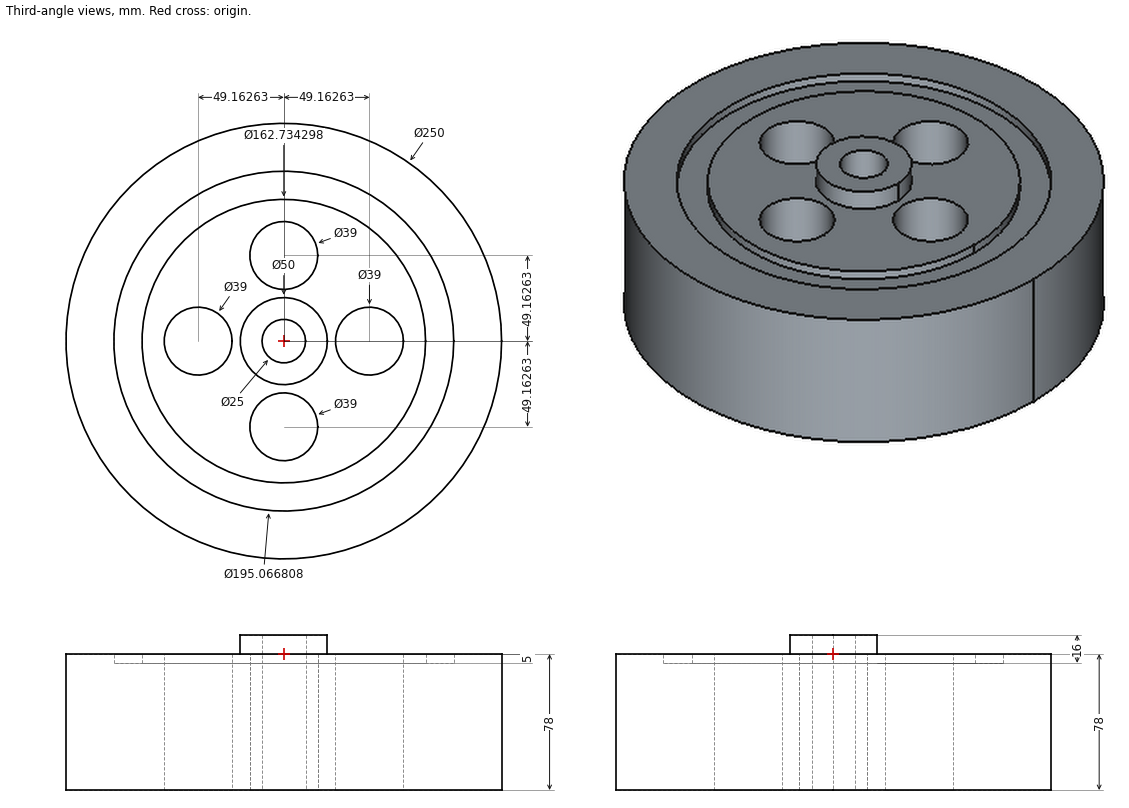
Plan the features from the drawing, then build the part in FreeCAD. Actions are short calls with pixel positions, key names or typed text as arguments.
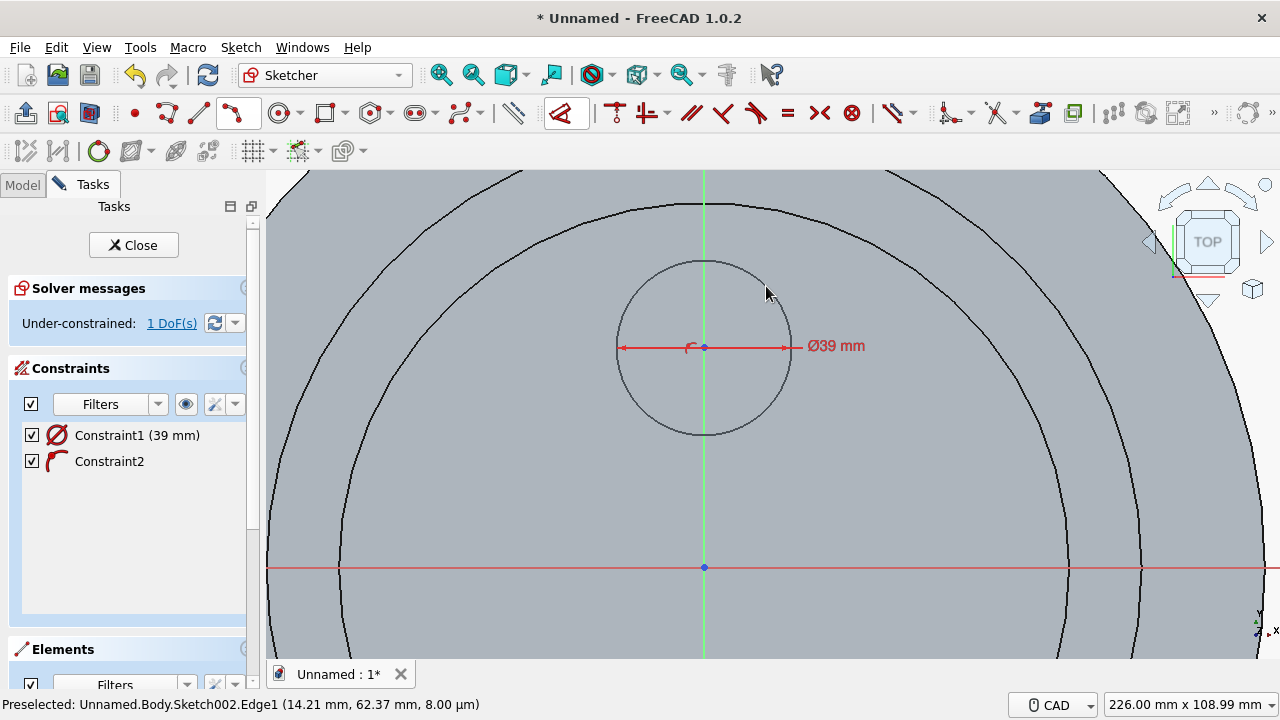
click(560, 114)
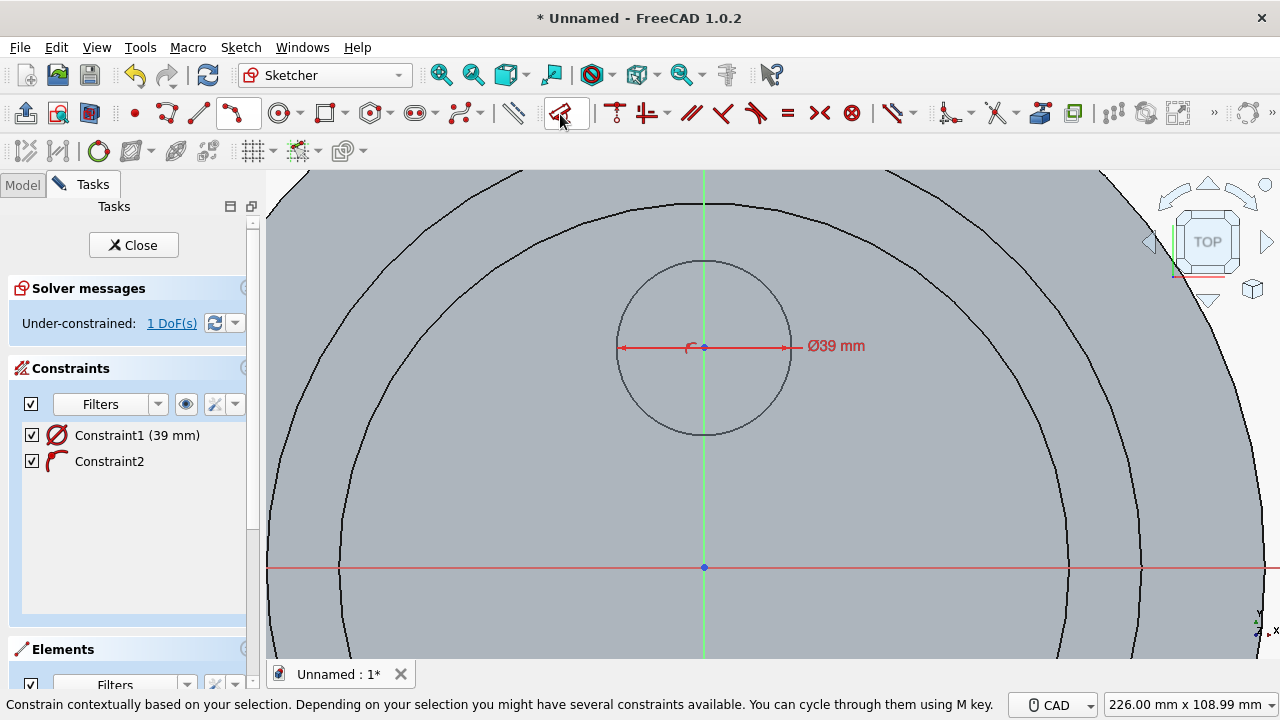
click(704, 348)
click(738, 458)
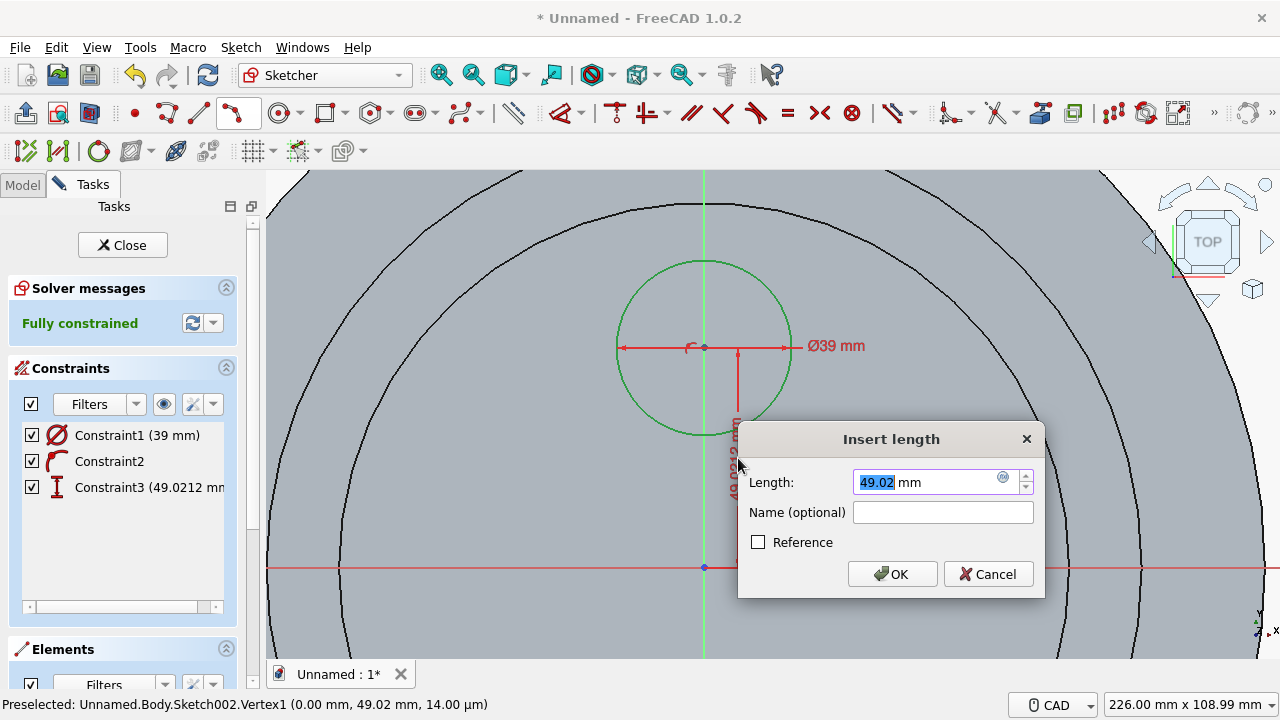
text(49.16263)
key(Return)
key(Escape)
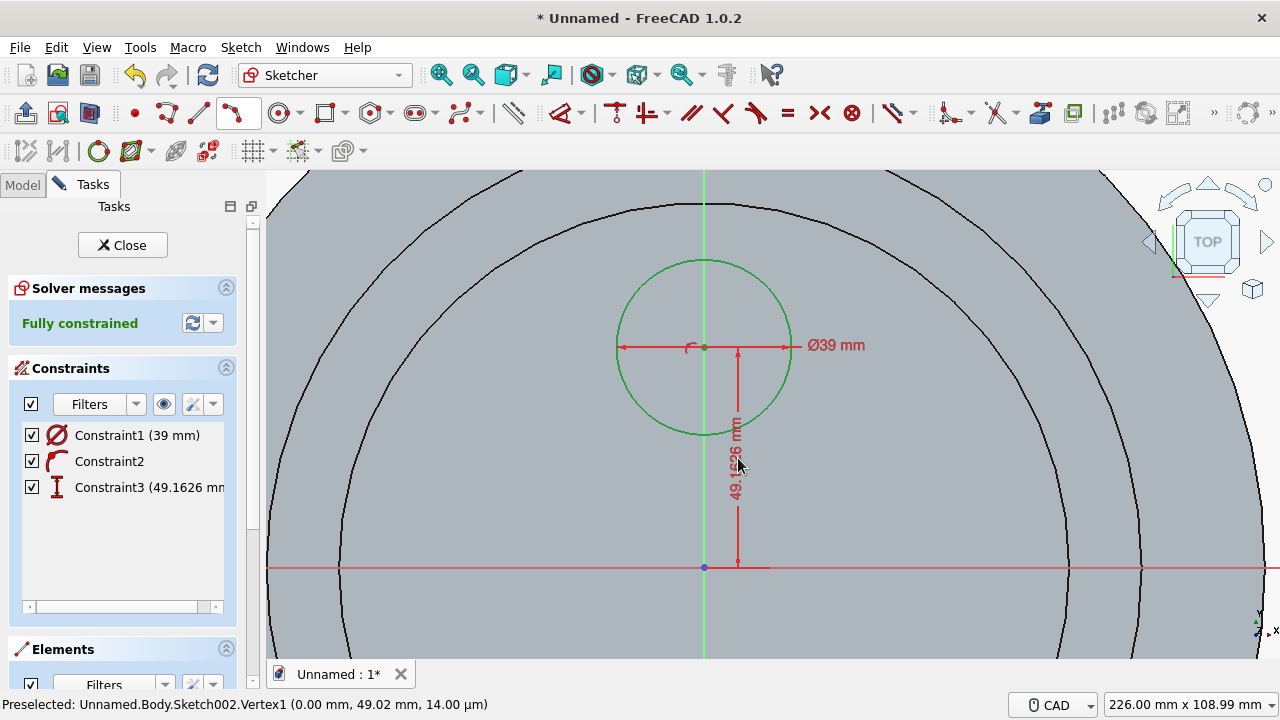
click(123, 245)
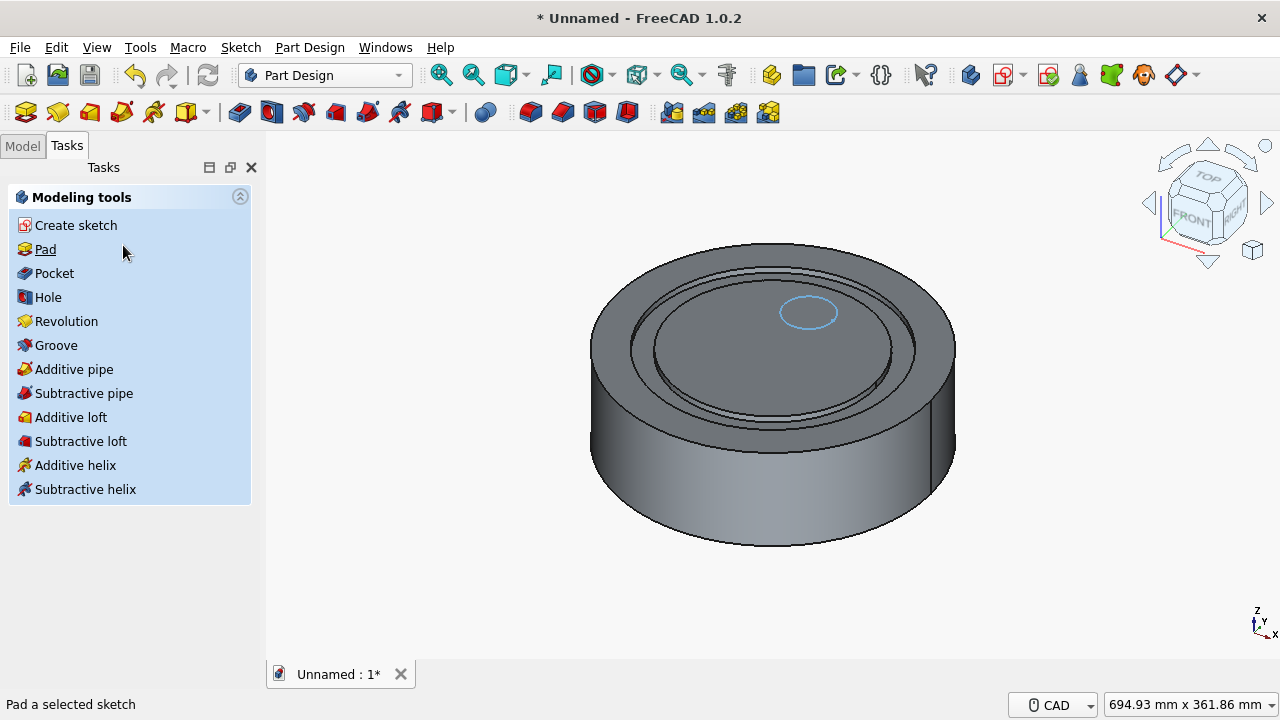
click(240, 112)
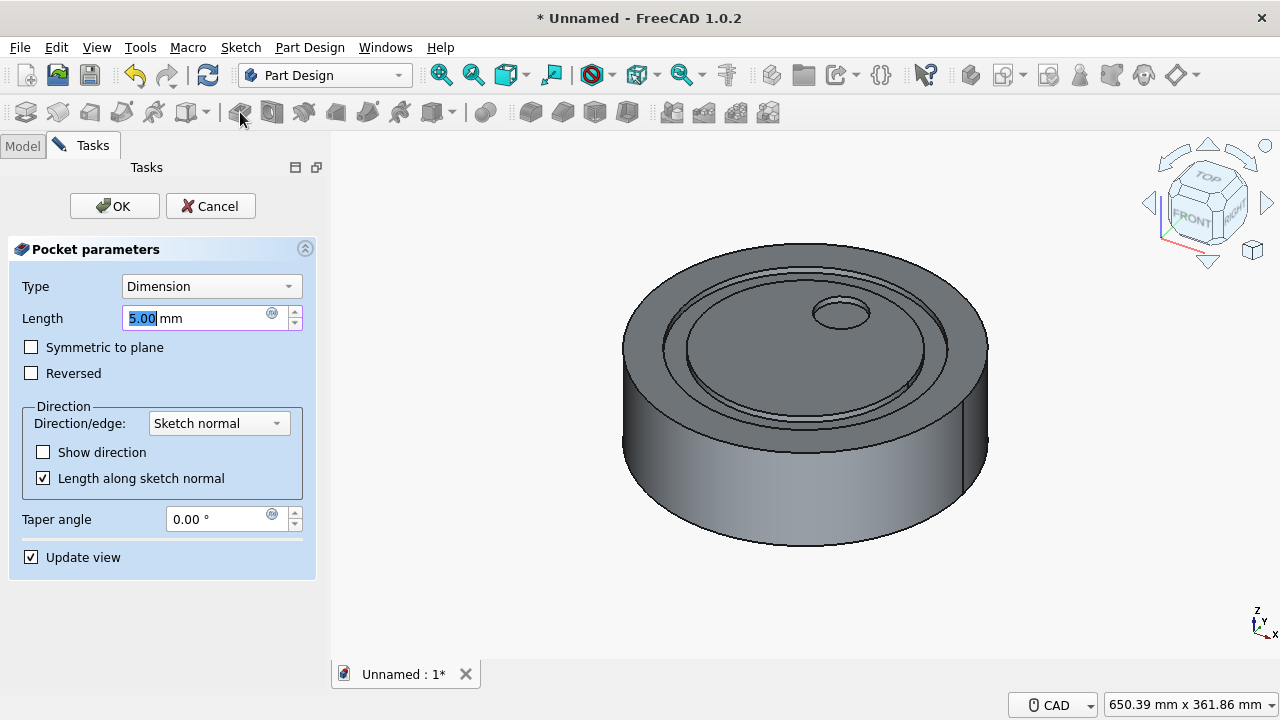
text(78)
key(Tab)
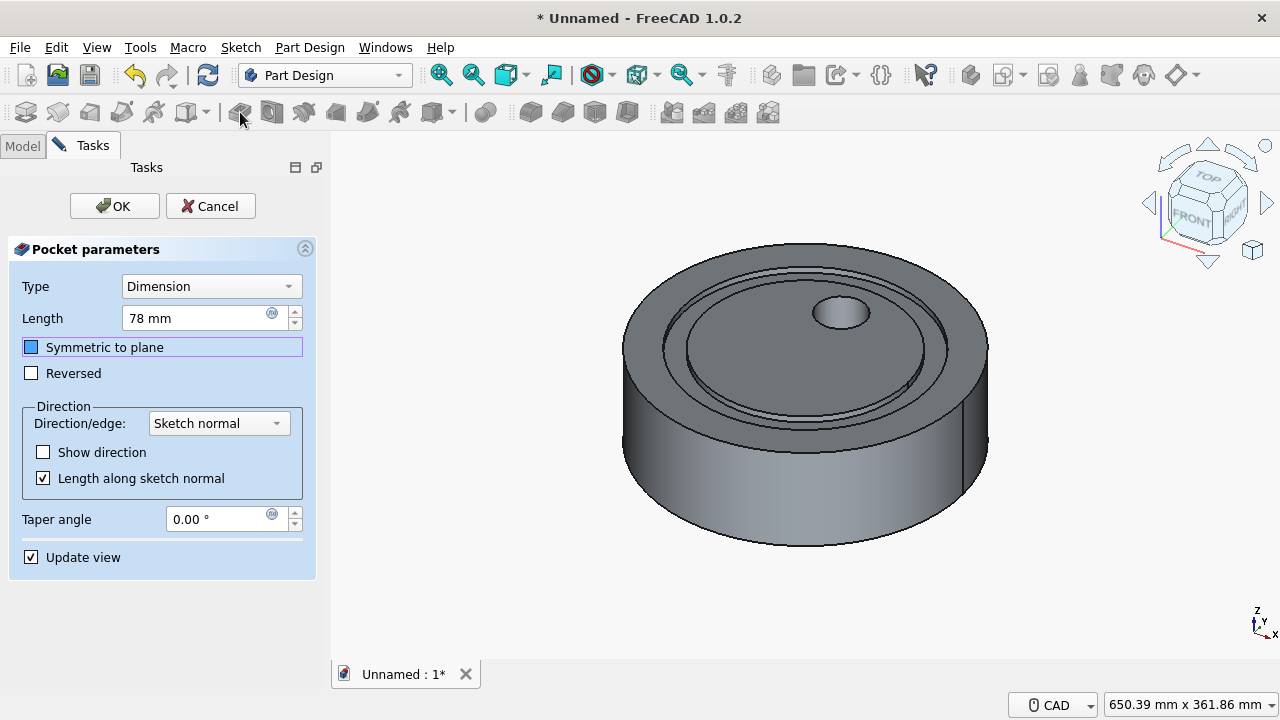
click(115, 206)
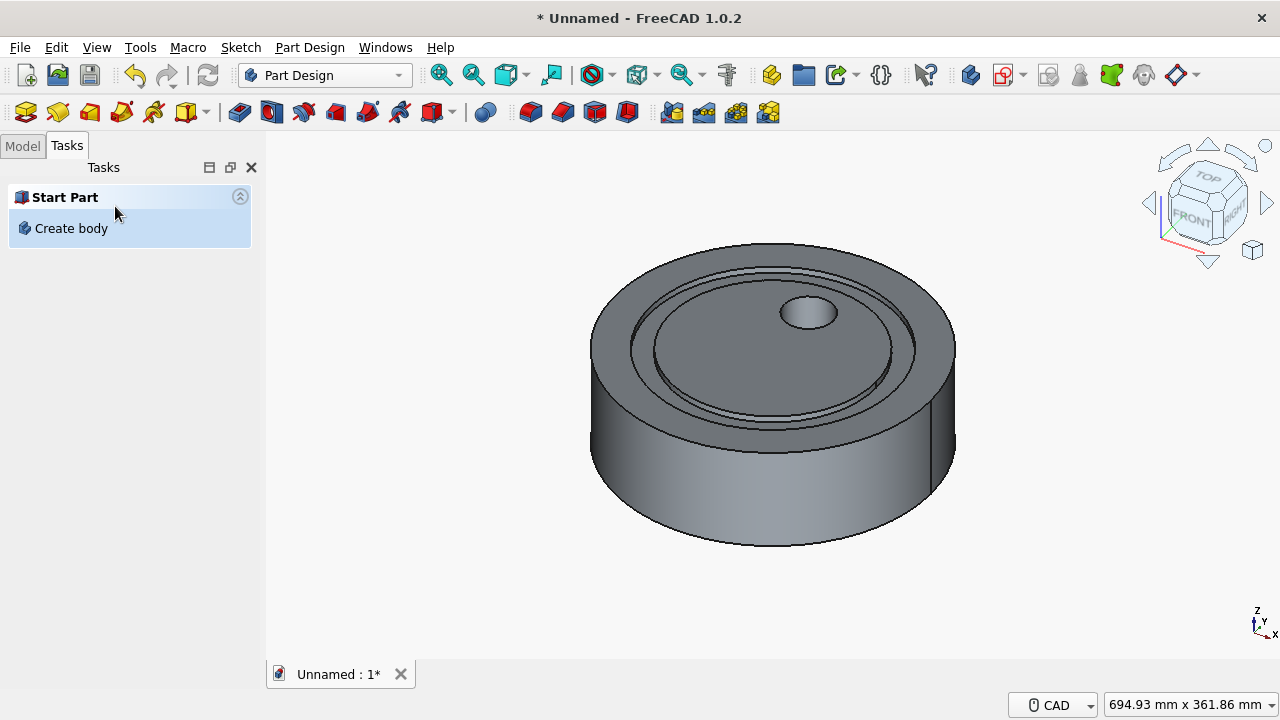
click(756, 364)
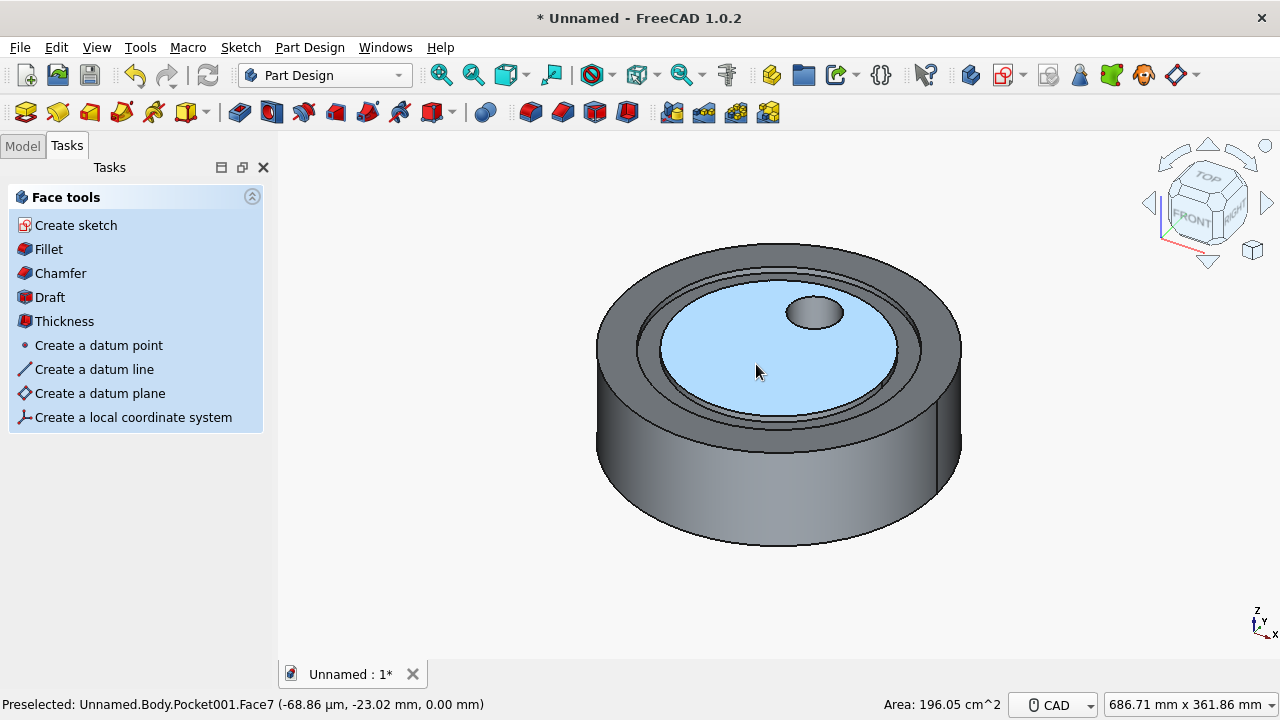
click(1004, 76)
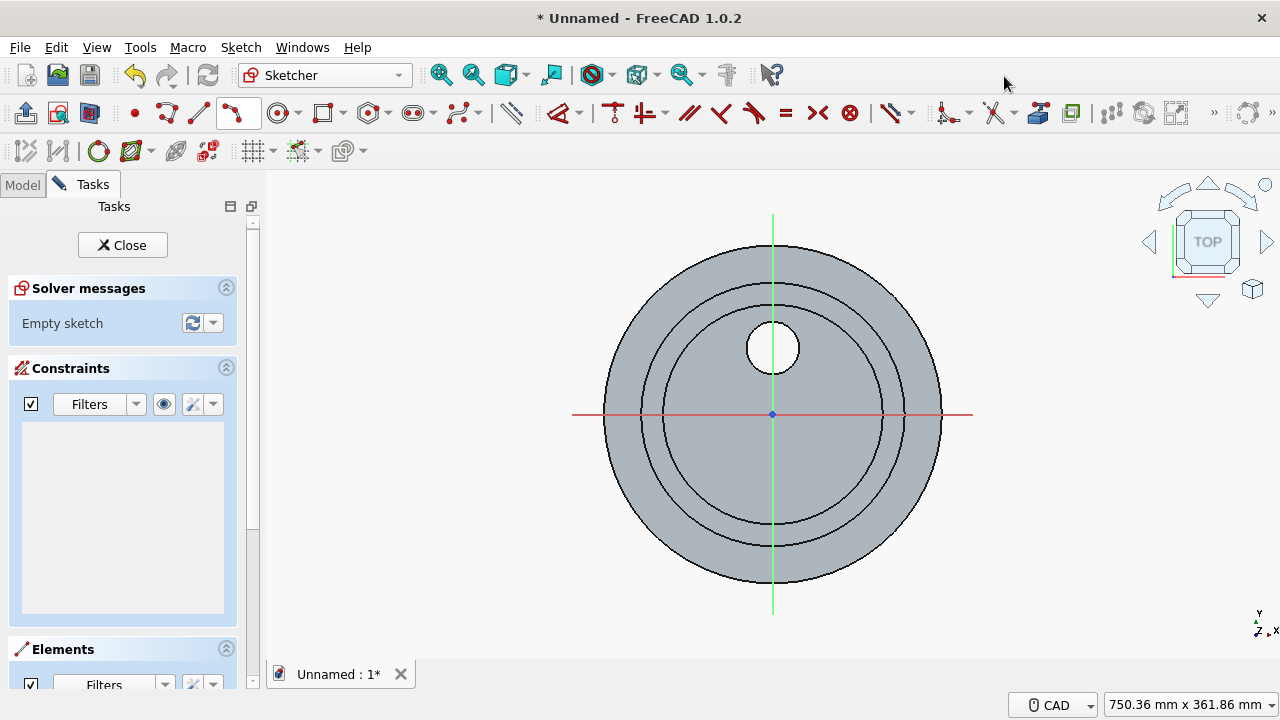
scroll(842, 414, up, 9)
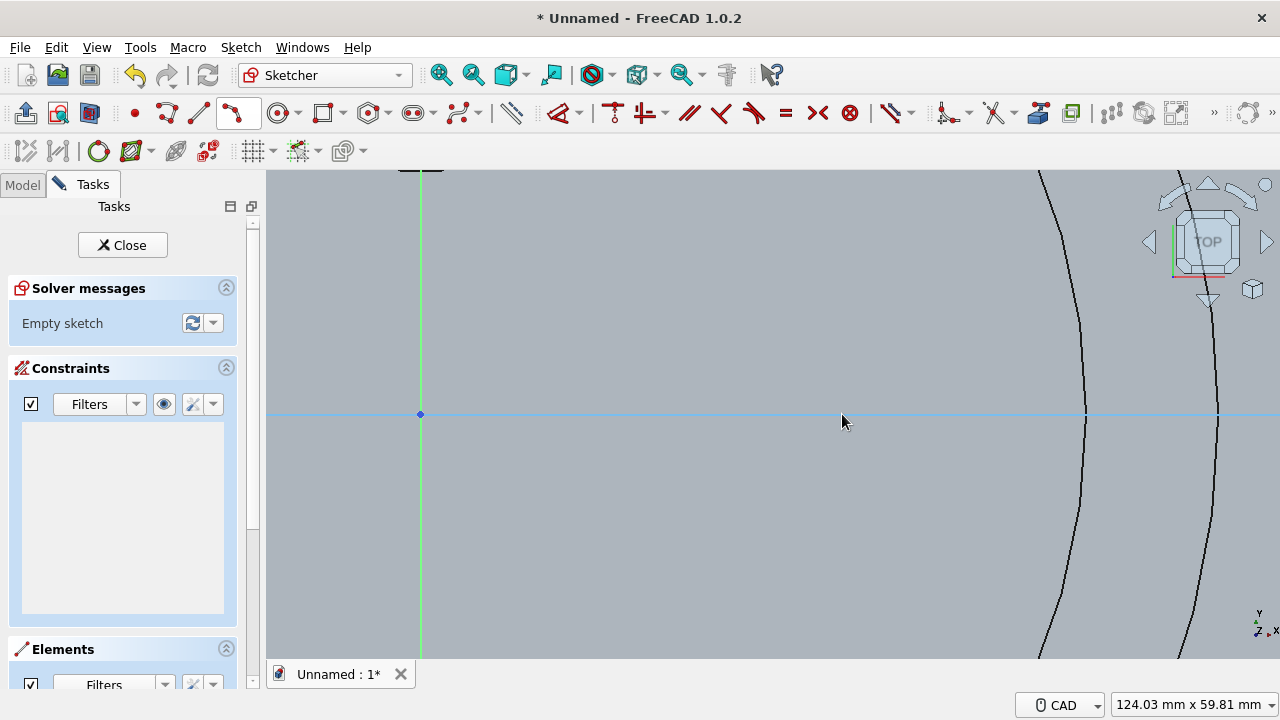
click(278, 114)